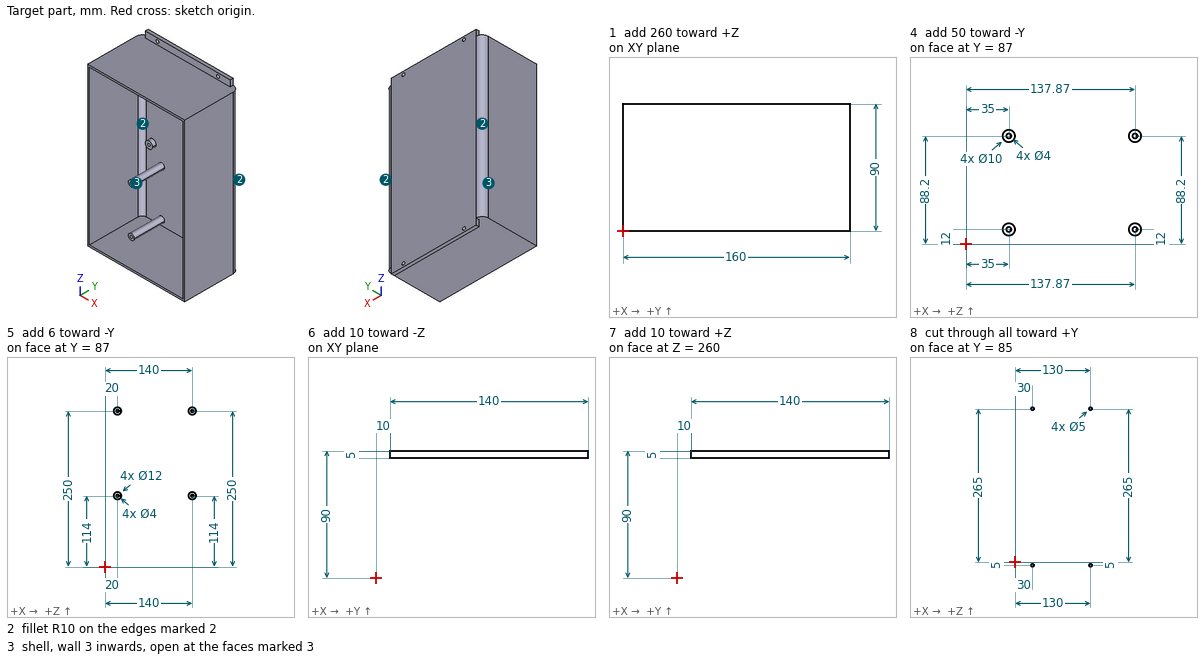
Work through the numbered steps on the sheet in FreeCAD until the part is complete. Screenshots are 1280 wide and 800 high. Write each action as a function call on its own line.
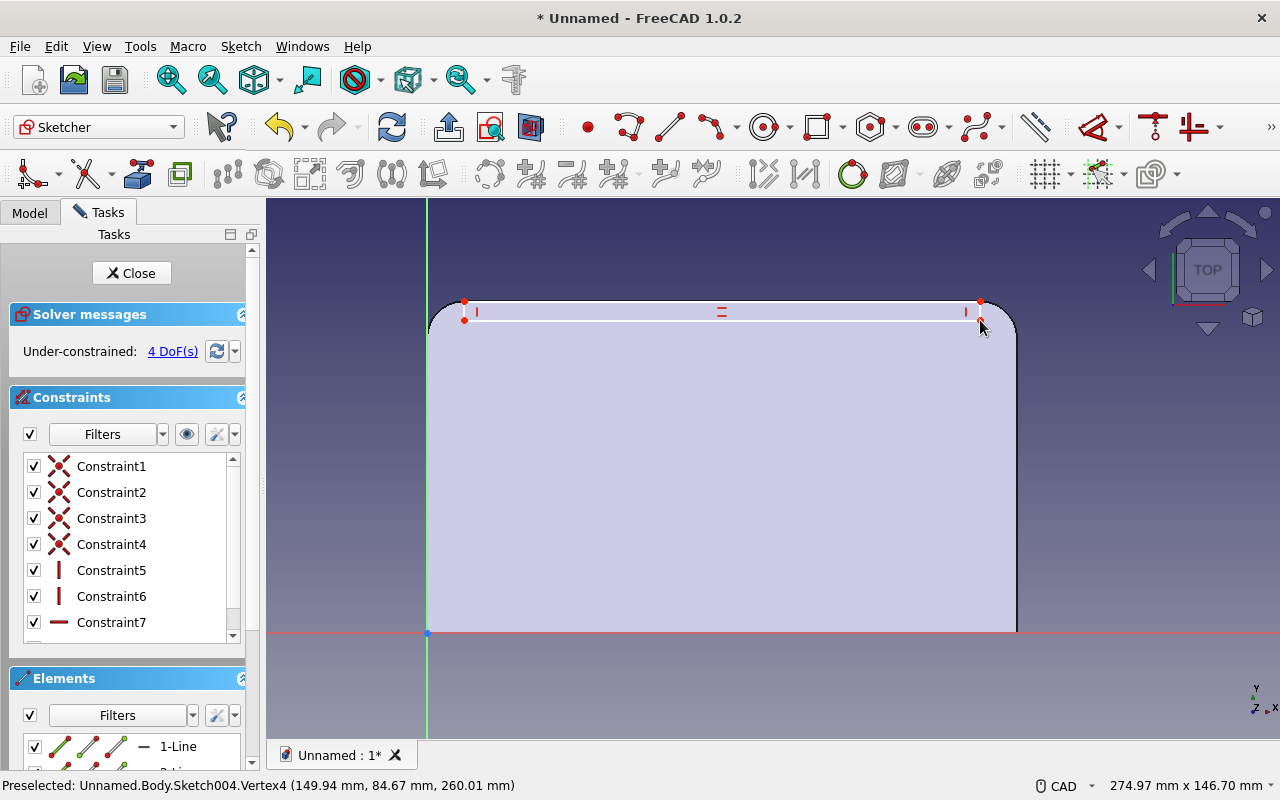
click(1092, 128)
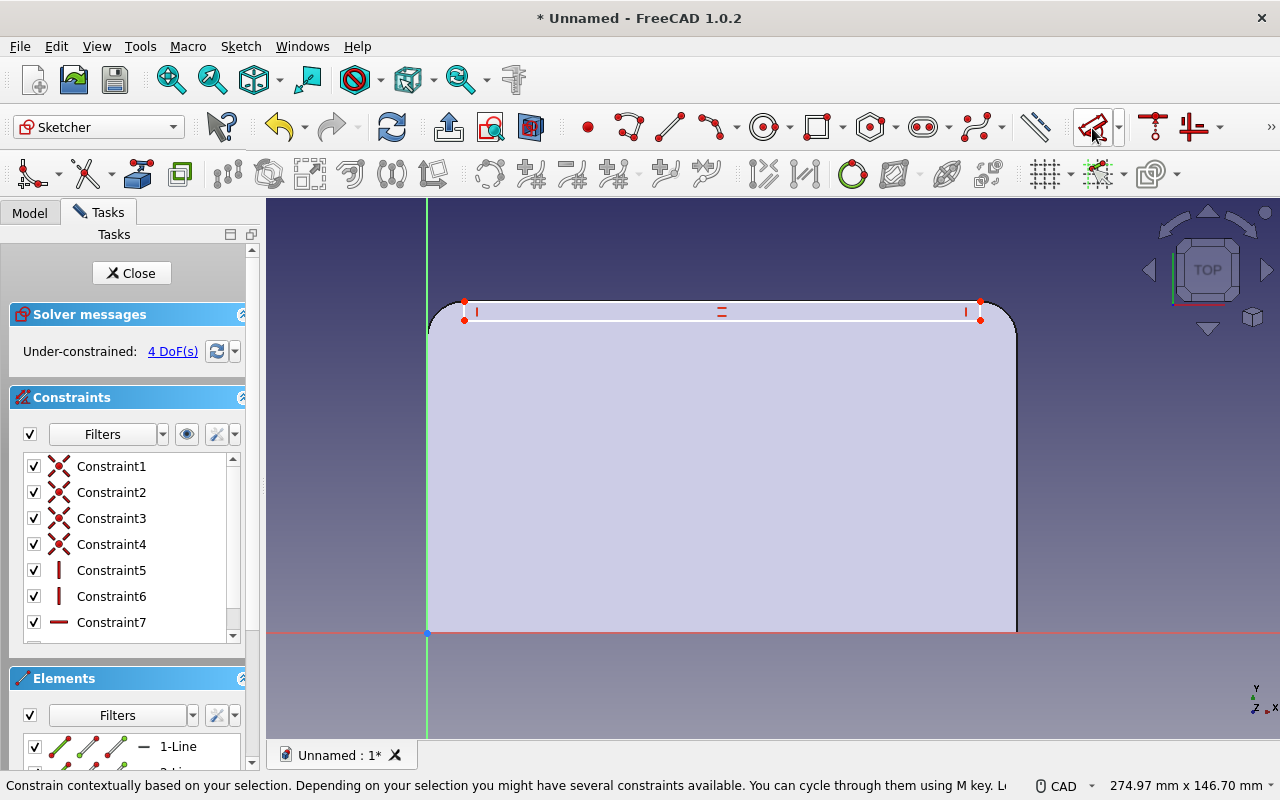
scroll(464, 312, up, 4)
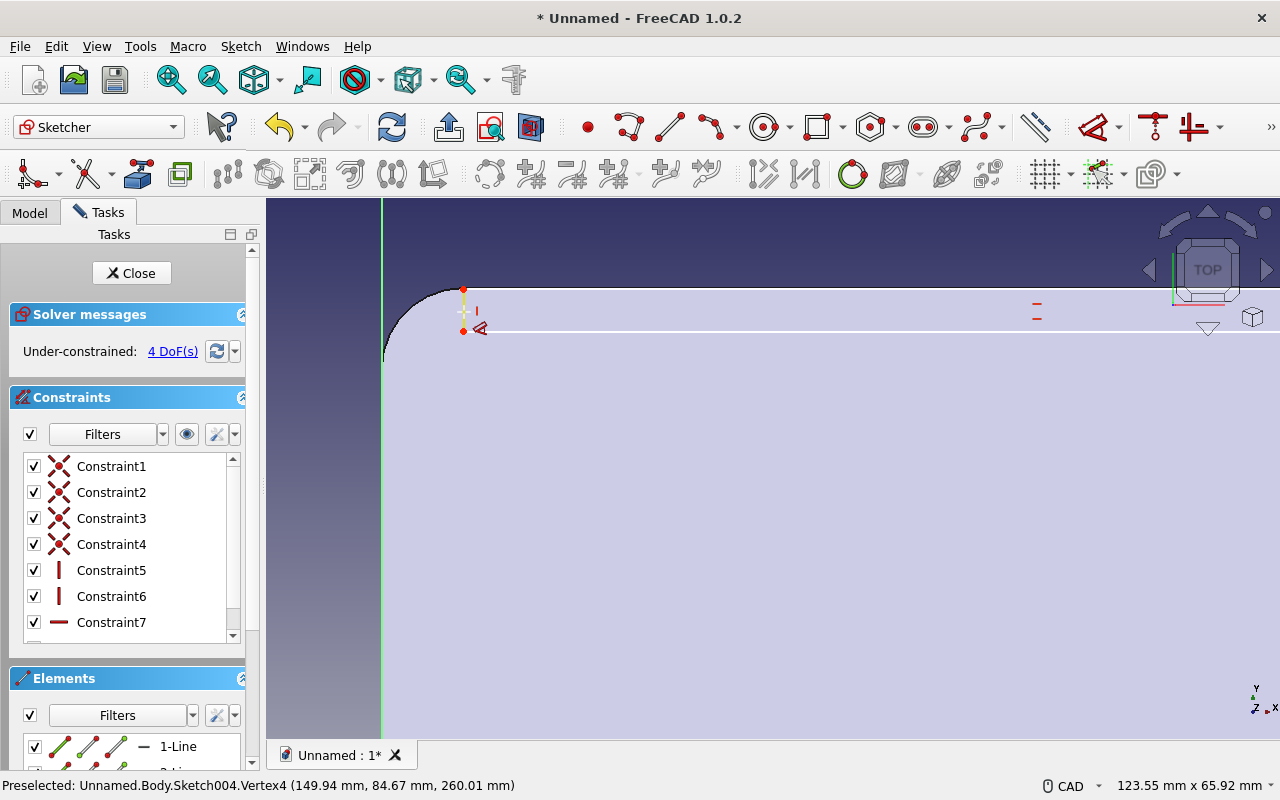
click(464, 311)
click(430, 311)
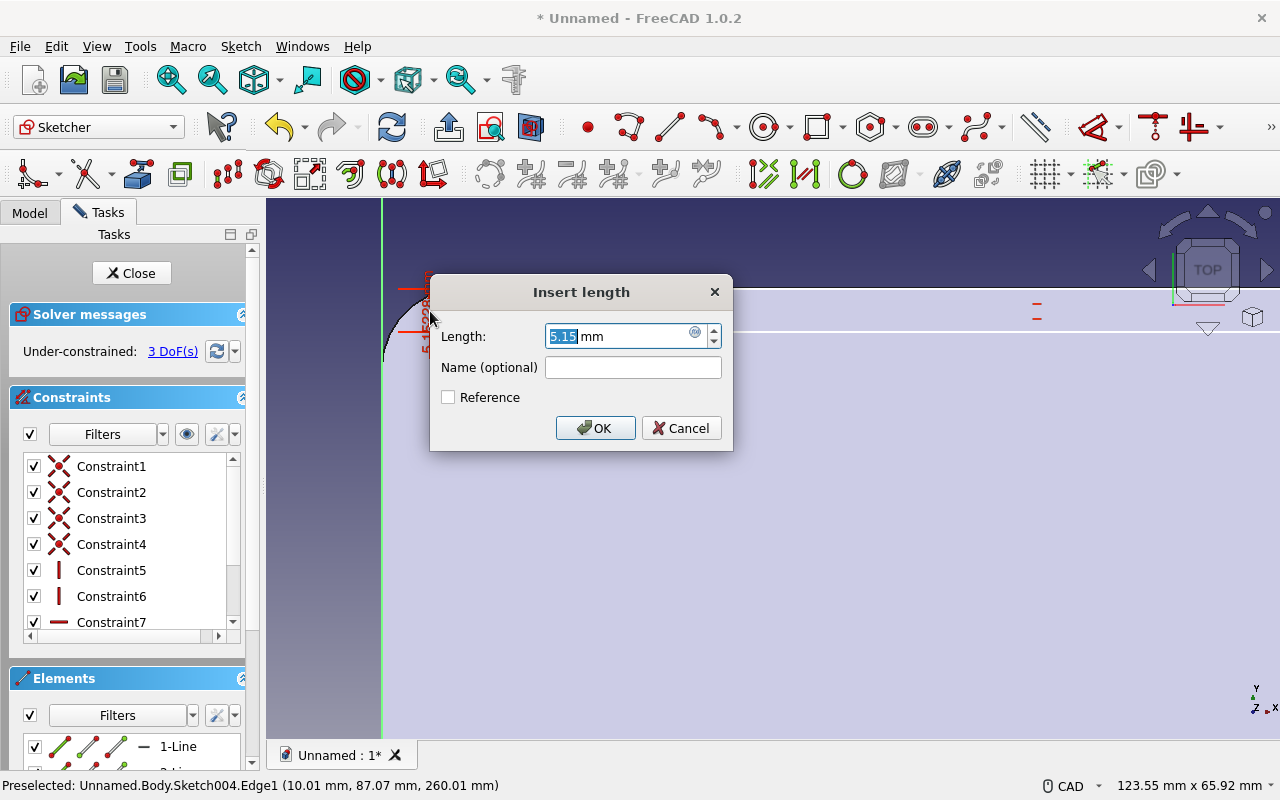
text(5)
key(Return)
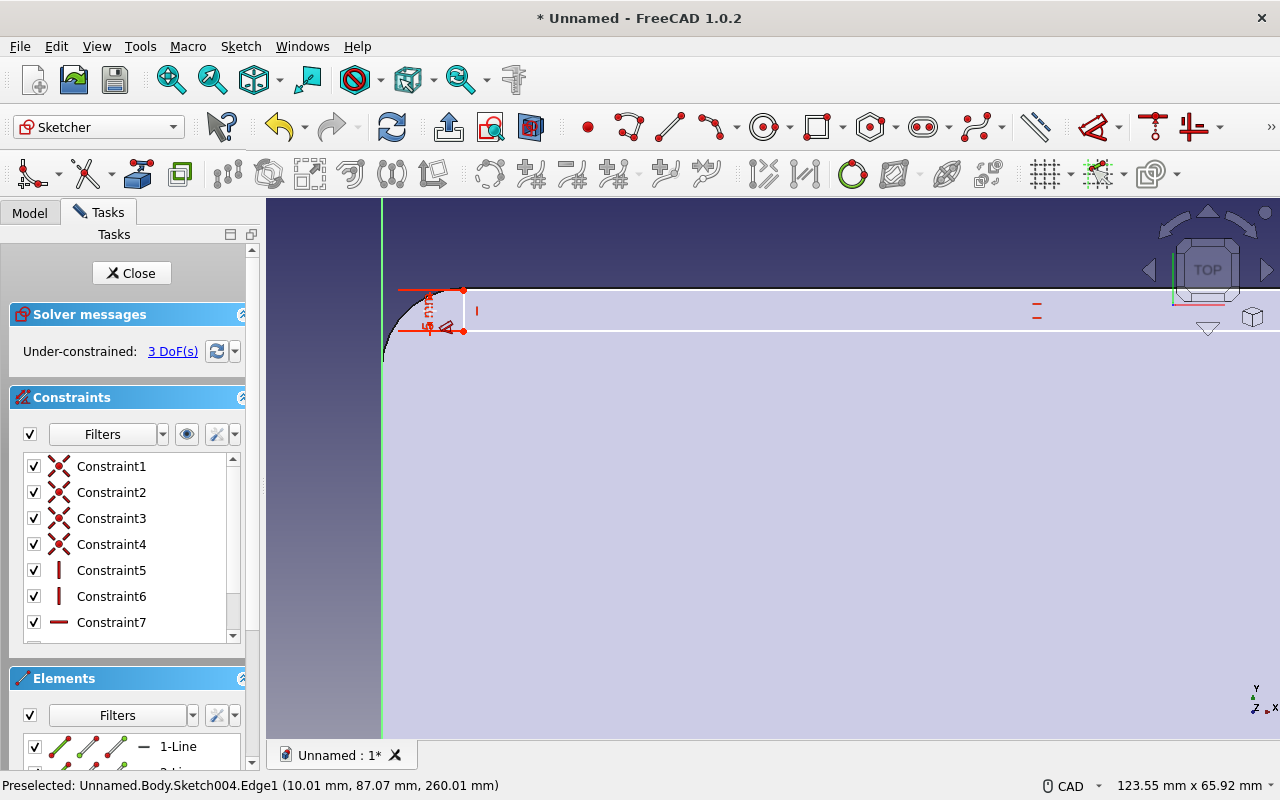
click(808, 331)
click(789, 365)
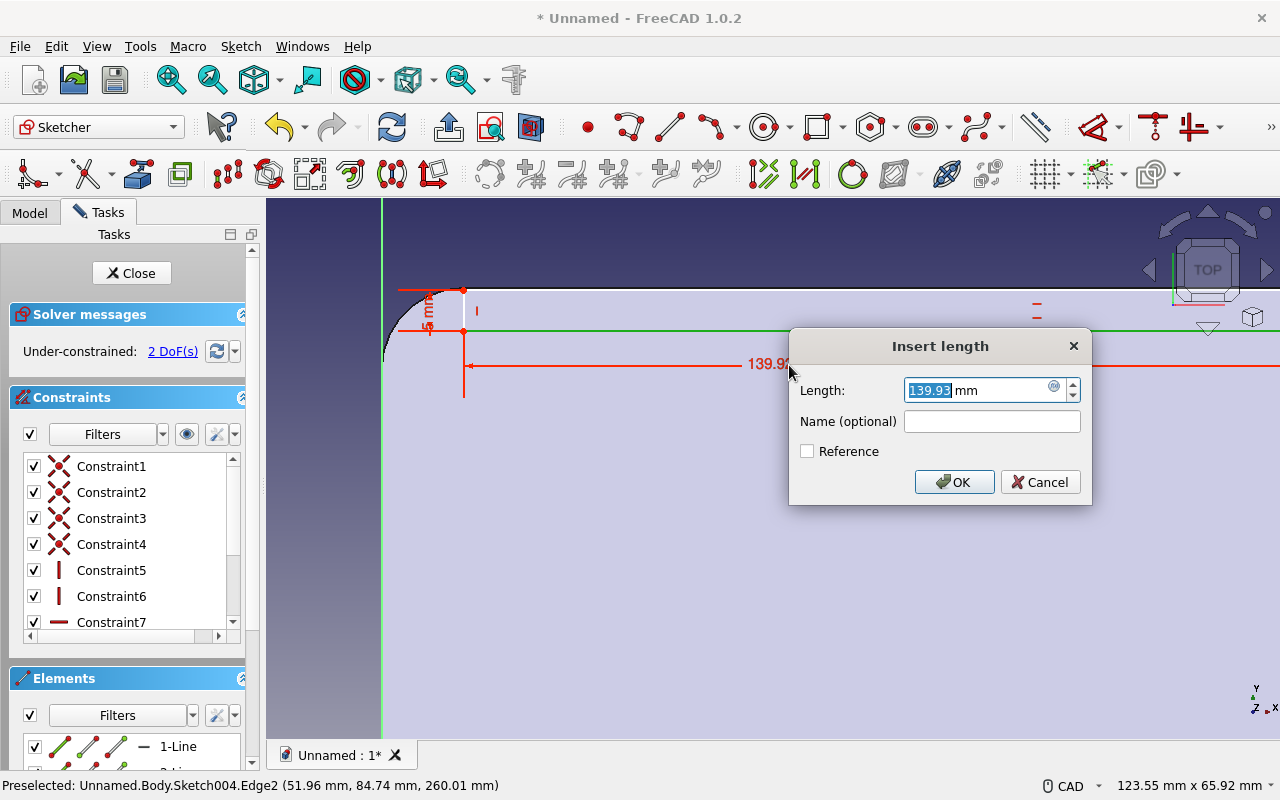
text(140)
key(Return)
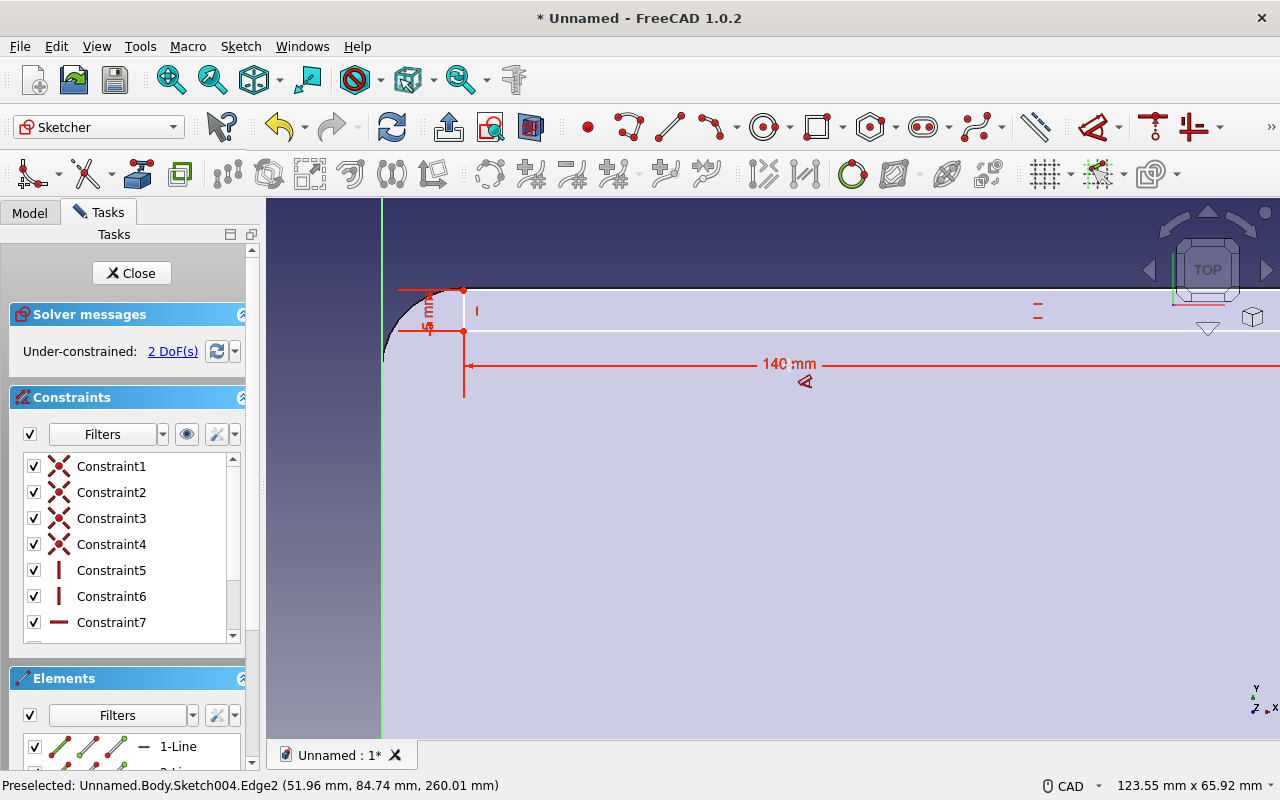
click(464, 290)
click(423, 256)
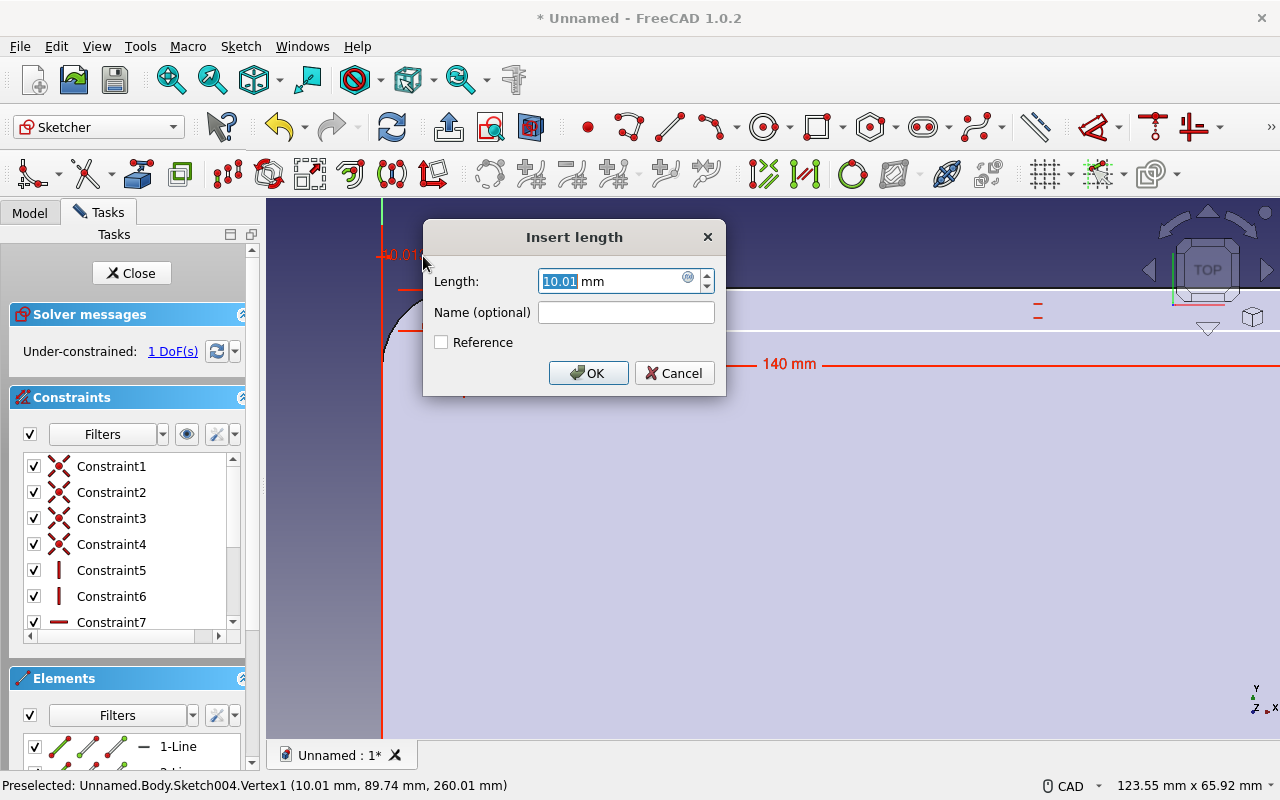
text(10)
key(Return)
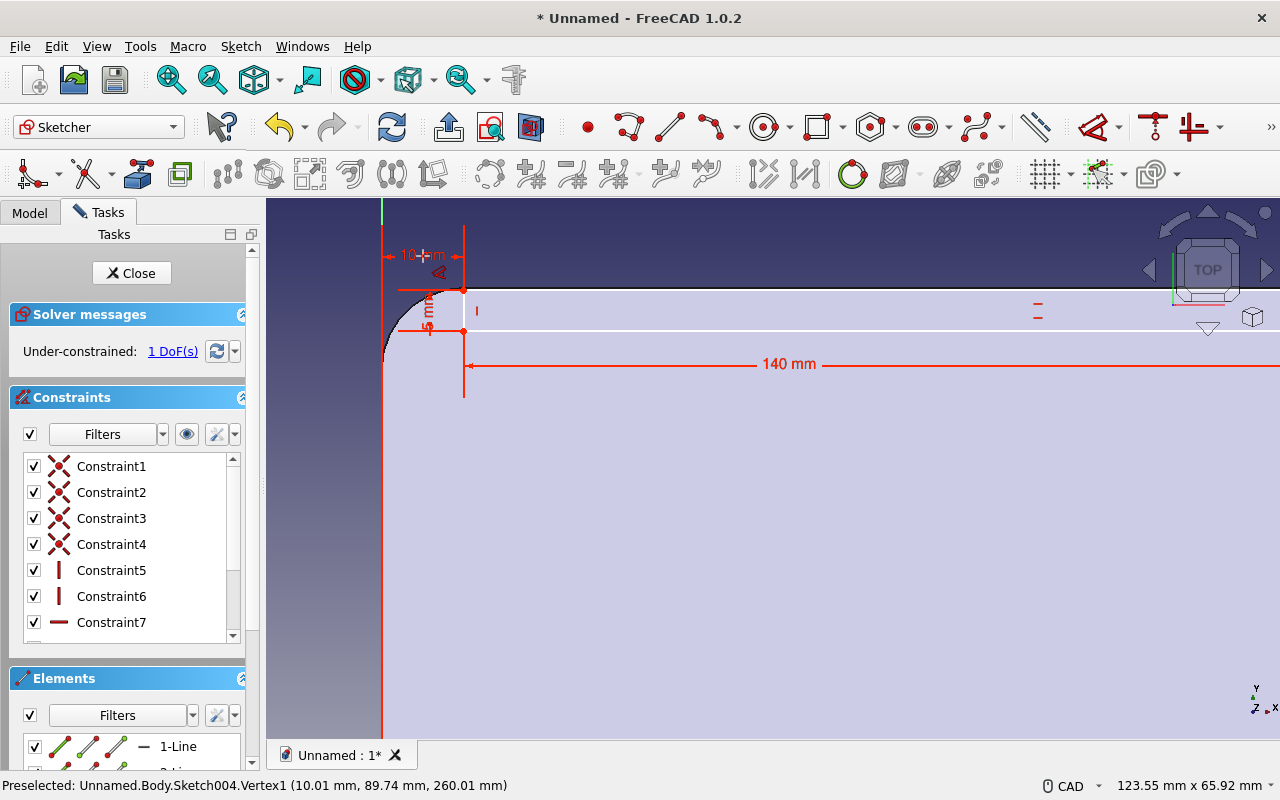
click(464, 290)
click(348, 501)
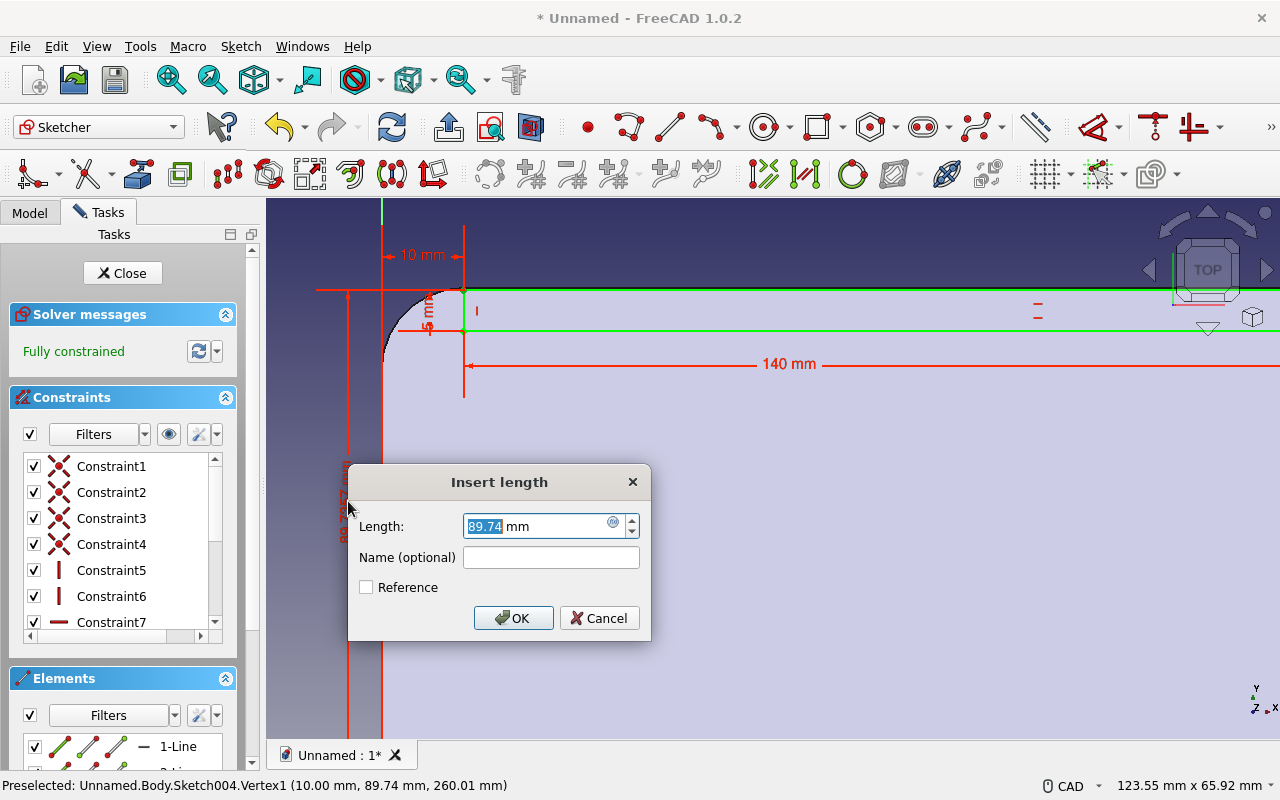
text(90)
key(Return)
key(Escape)